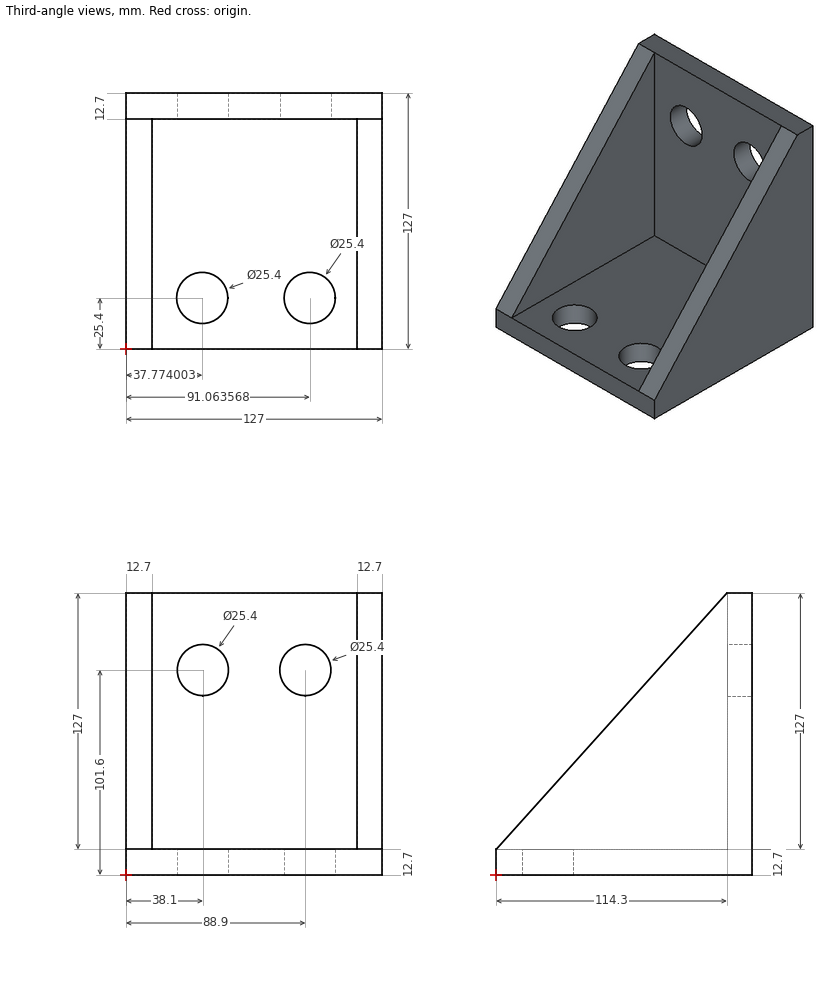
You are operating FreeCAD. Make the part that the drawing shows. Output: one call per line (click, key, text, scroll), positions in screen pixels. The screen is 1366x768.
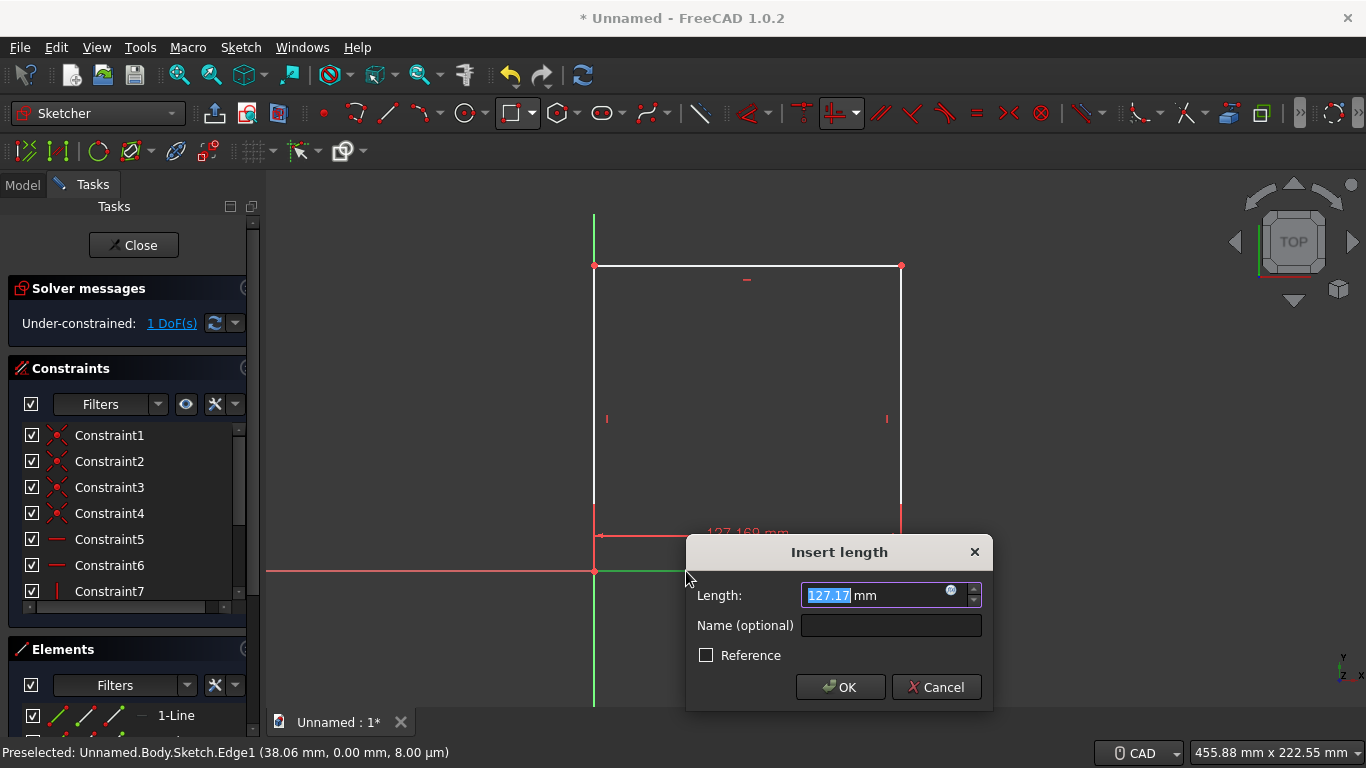
text(127)
key(Return)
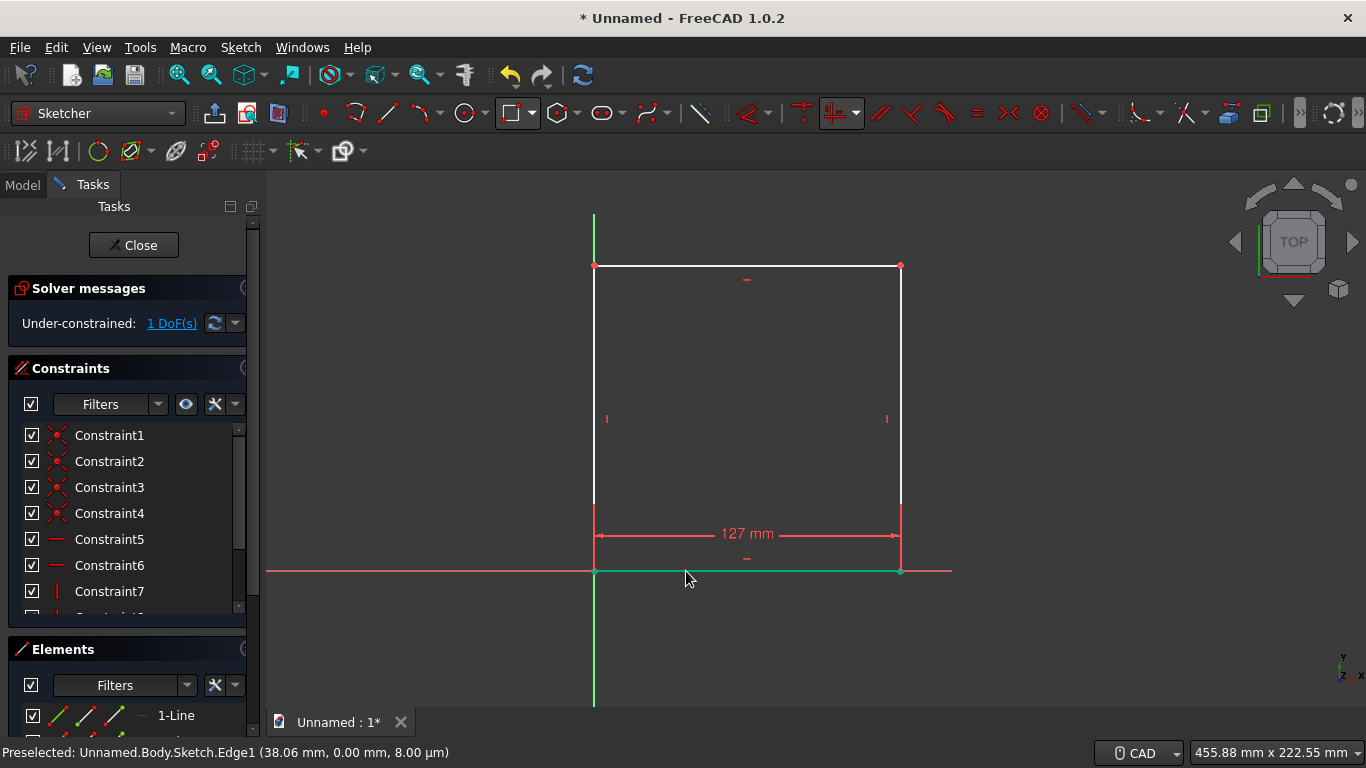
click(901, 480)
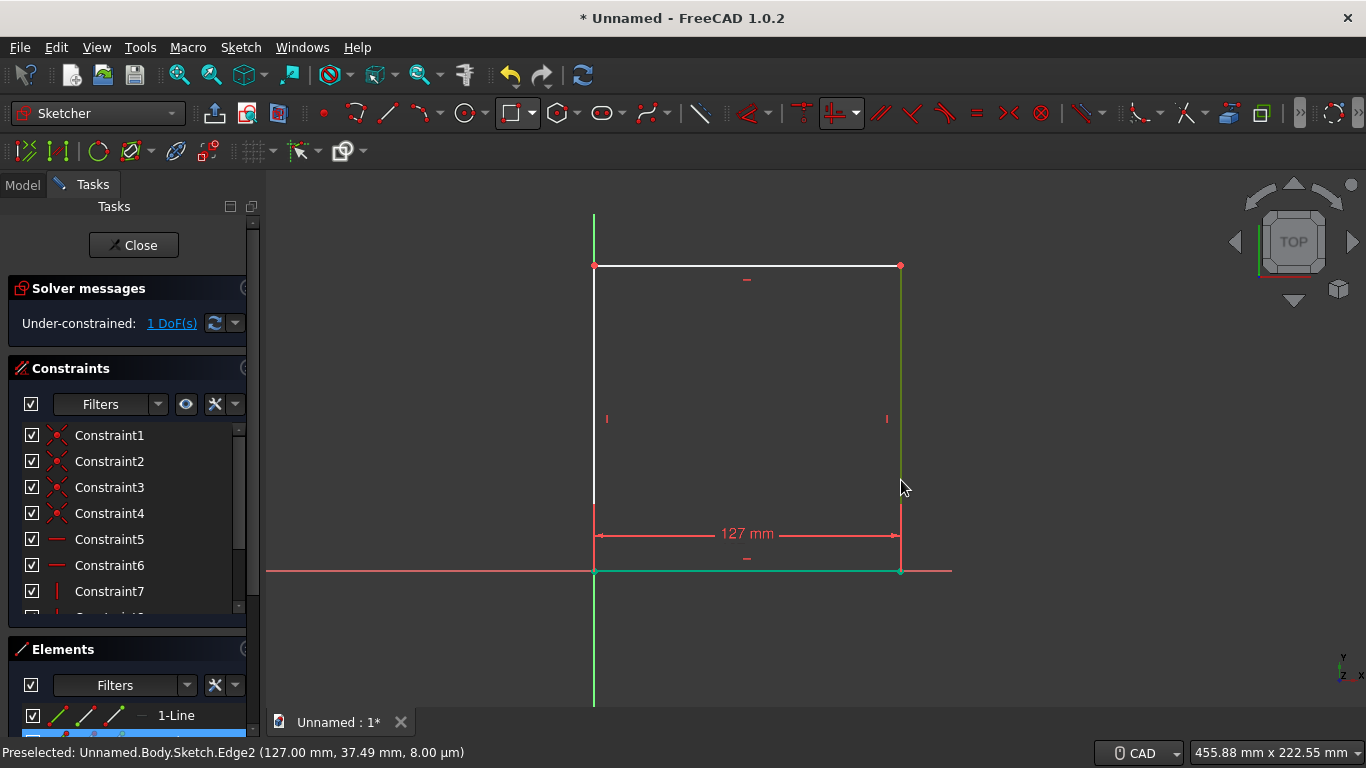
click(770, 114)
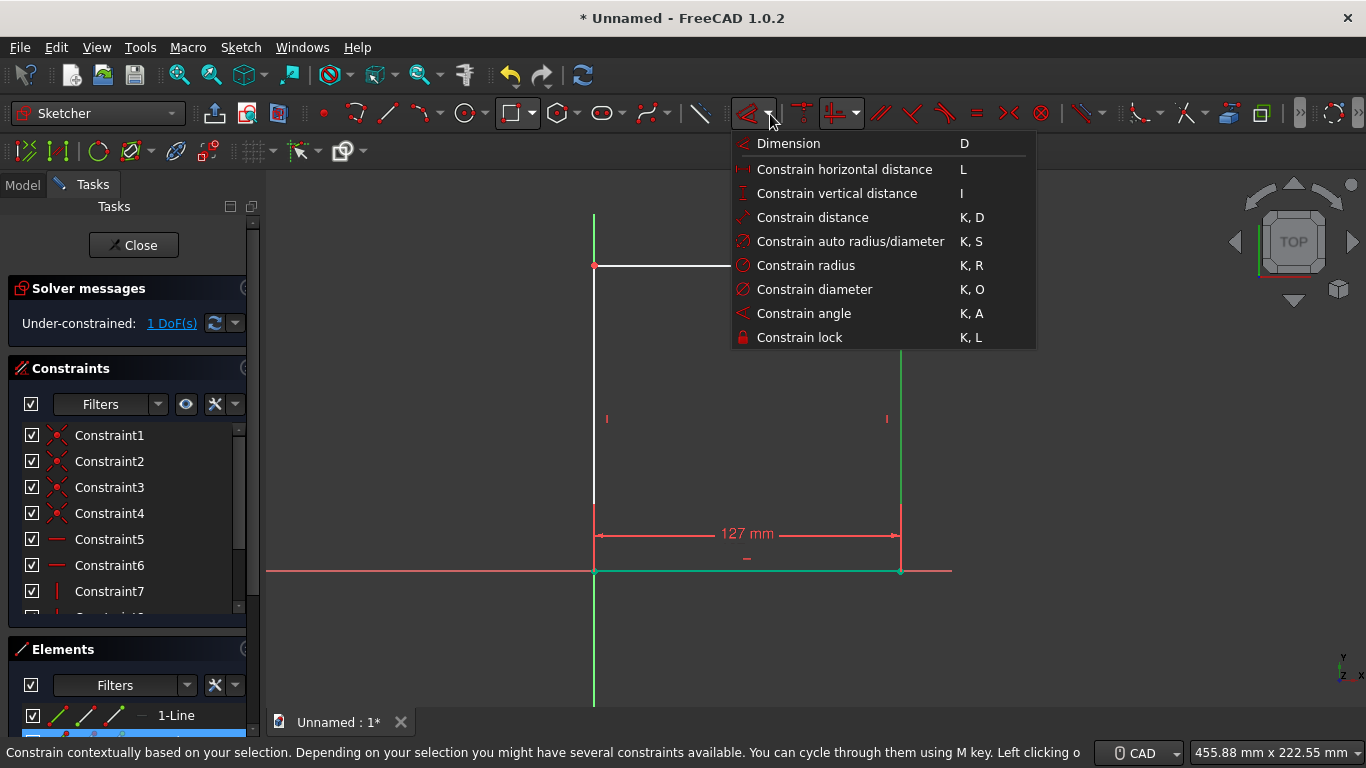
click(884, 193)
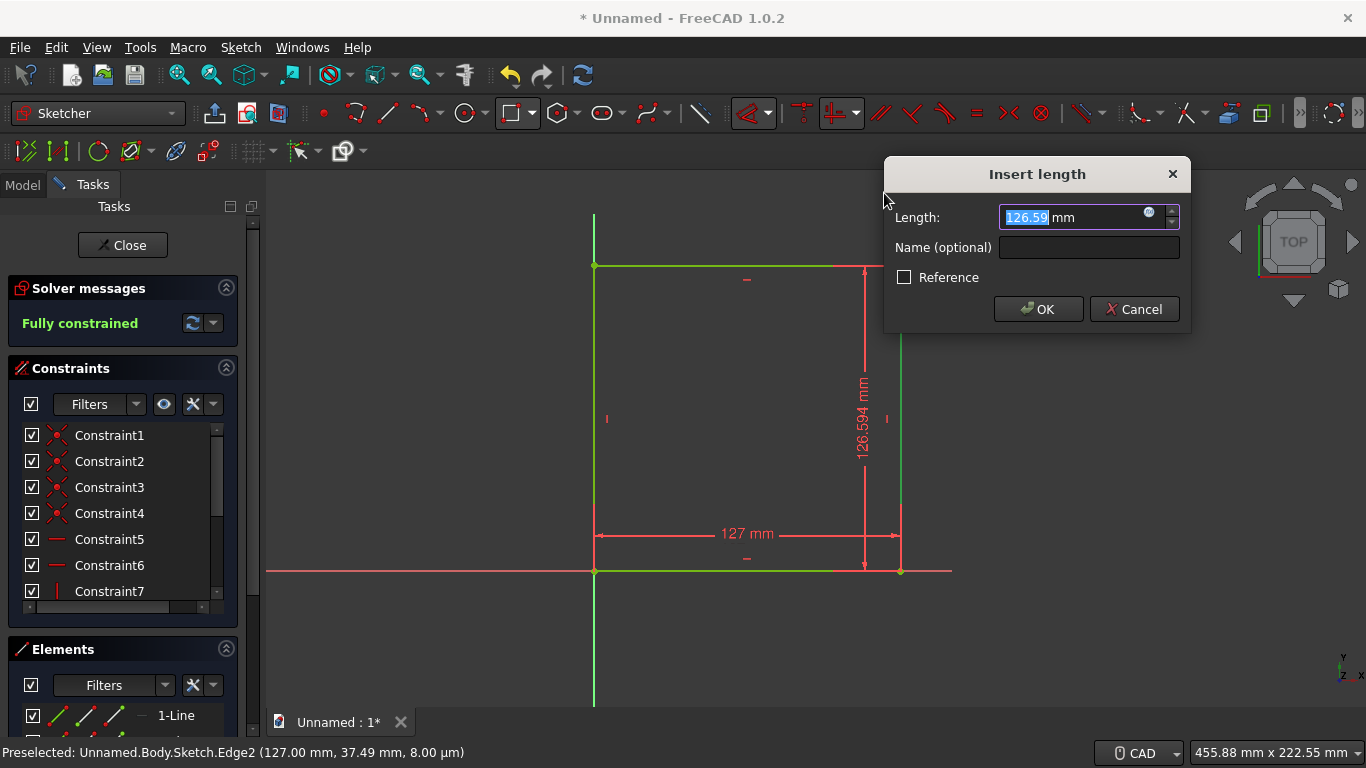
text(127)
key(Return)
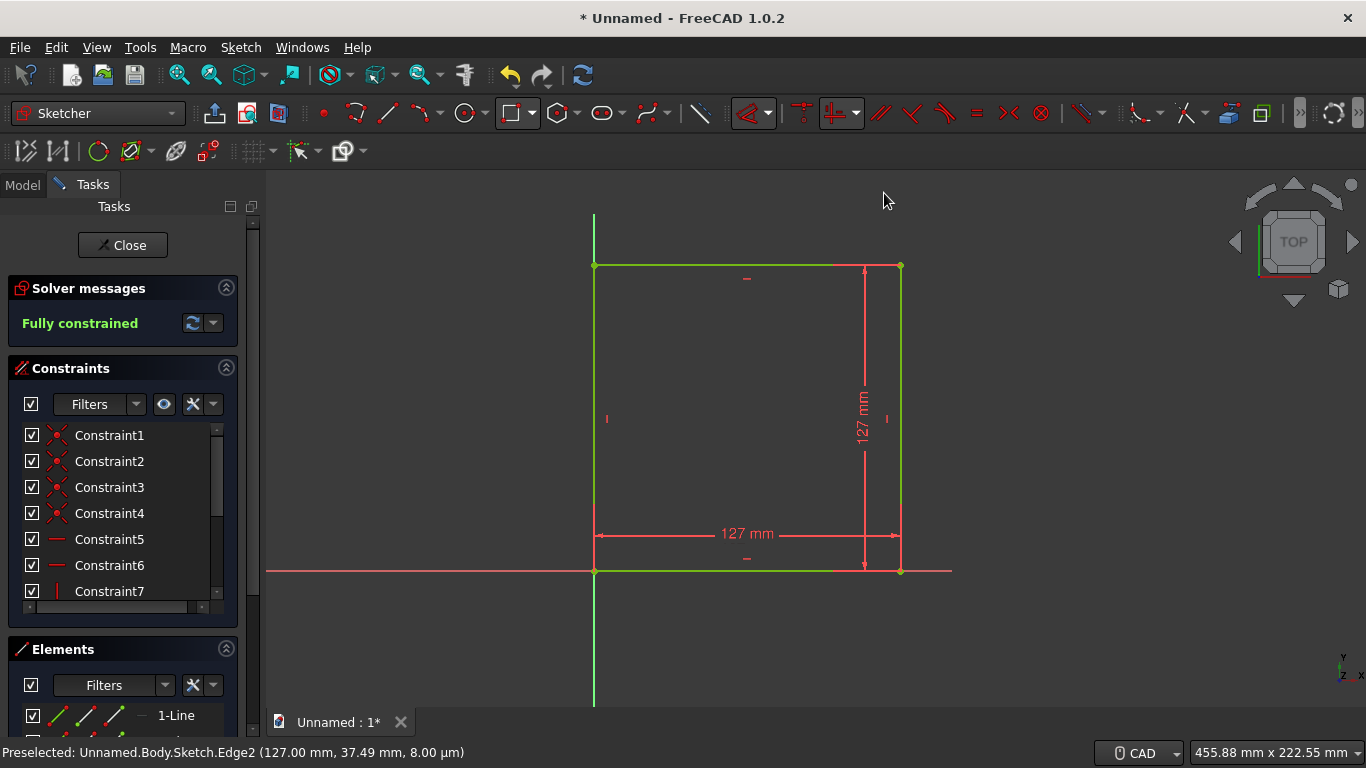
click(123, 245)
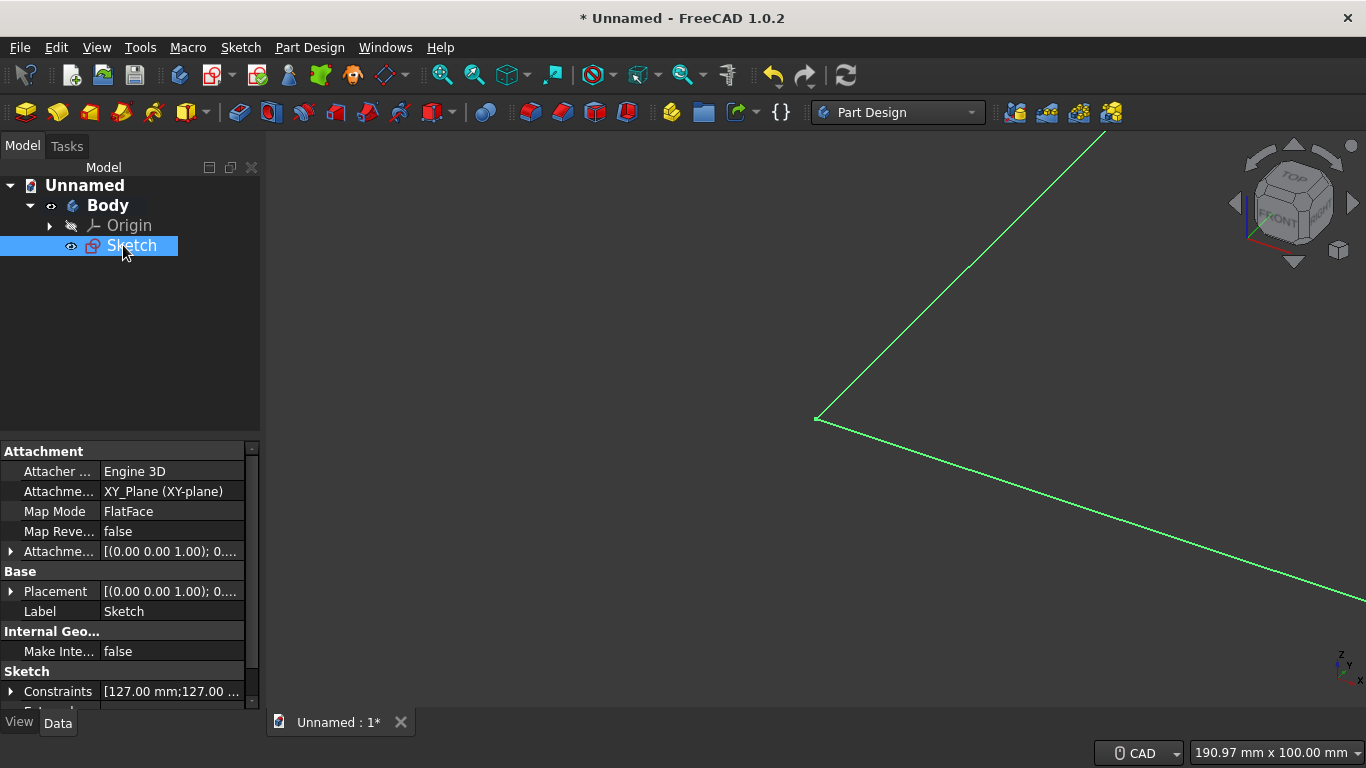
click(26, 112)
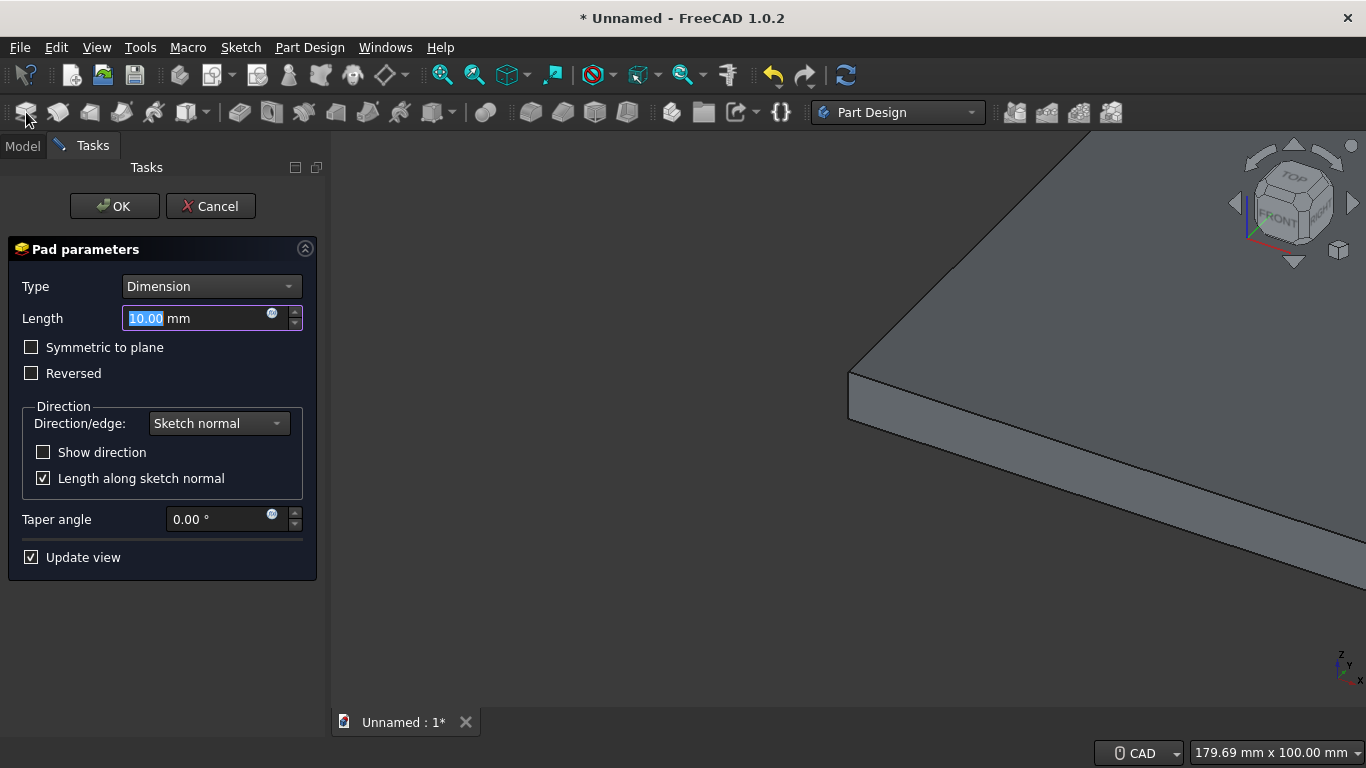
text(12.7)
key(Tab)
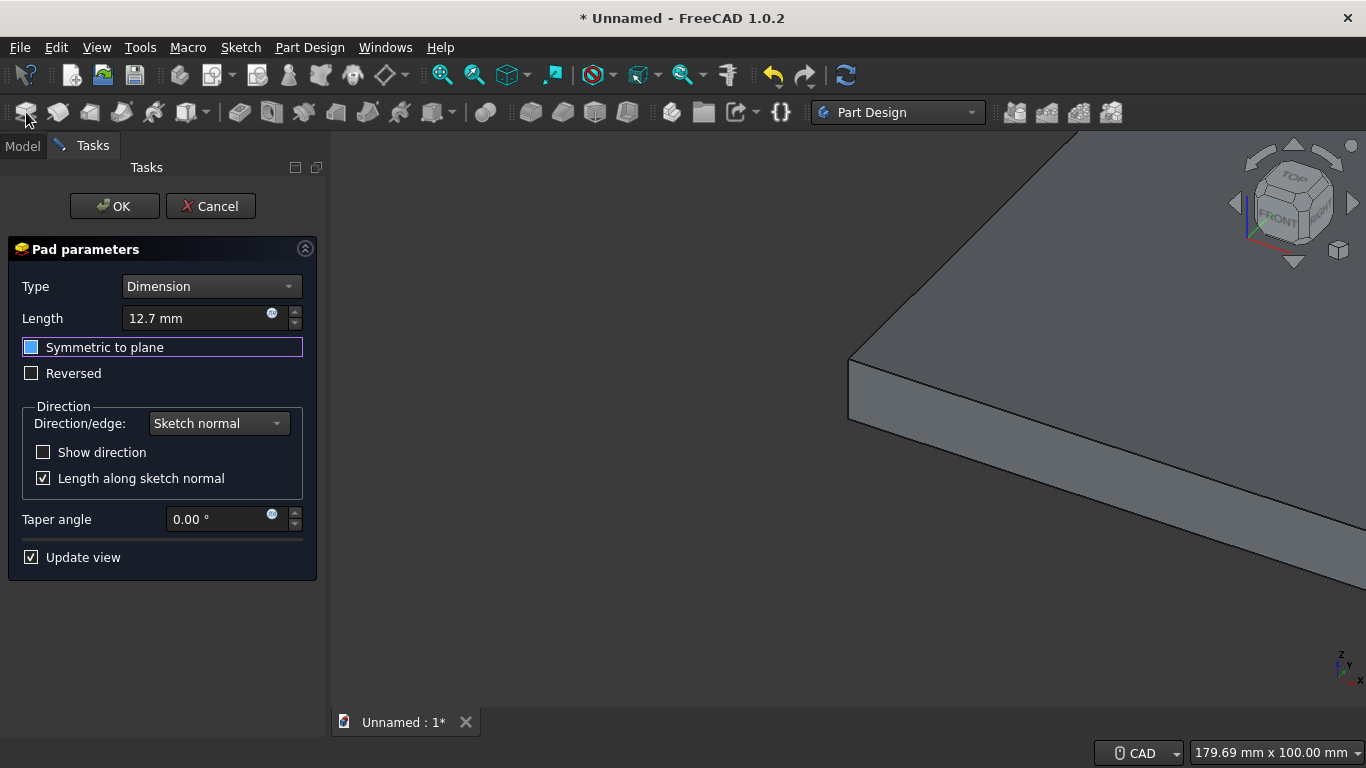
click(115, 206)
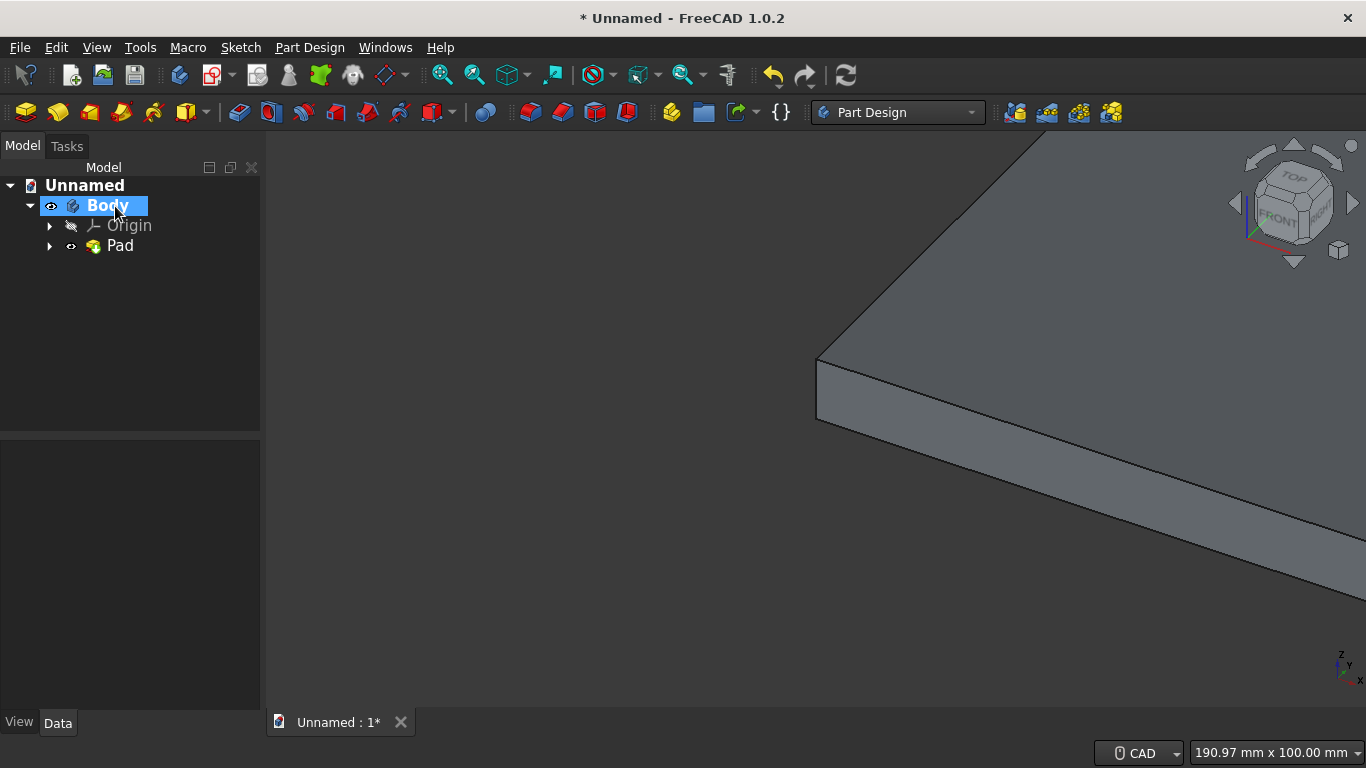
key(v)
key(f)